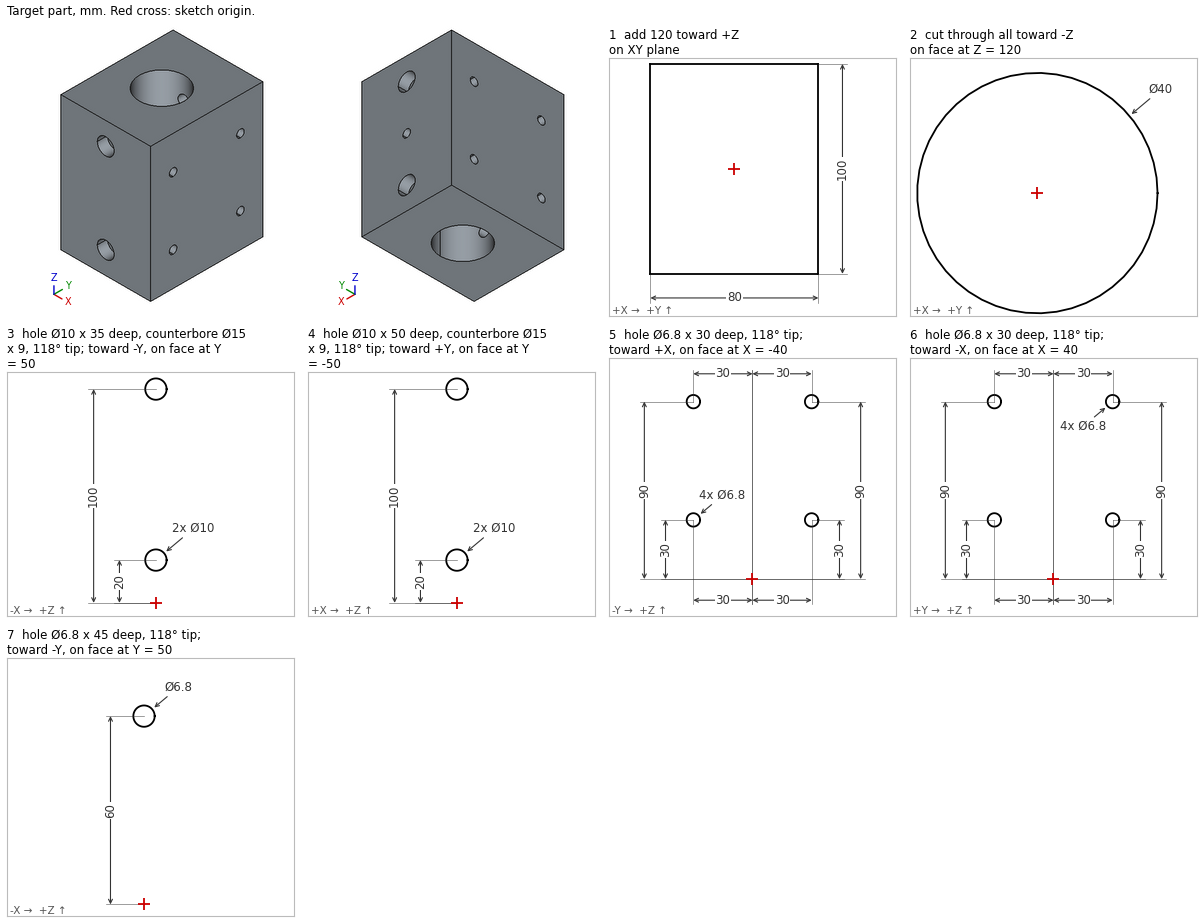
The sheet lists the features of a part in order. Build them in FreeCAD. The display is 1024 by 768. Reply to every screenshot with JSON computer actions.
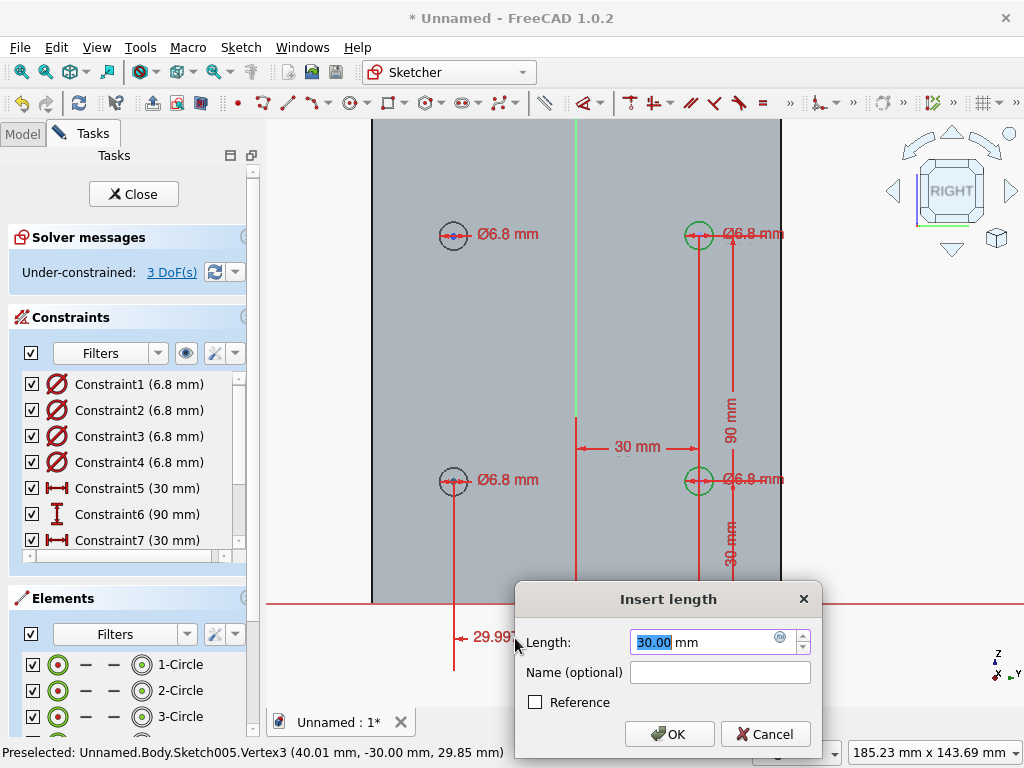
{"action": "type", "text": "30"}
{"action": "key", "text": "Return"}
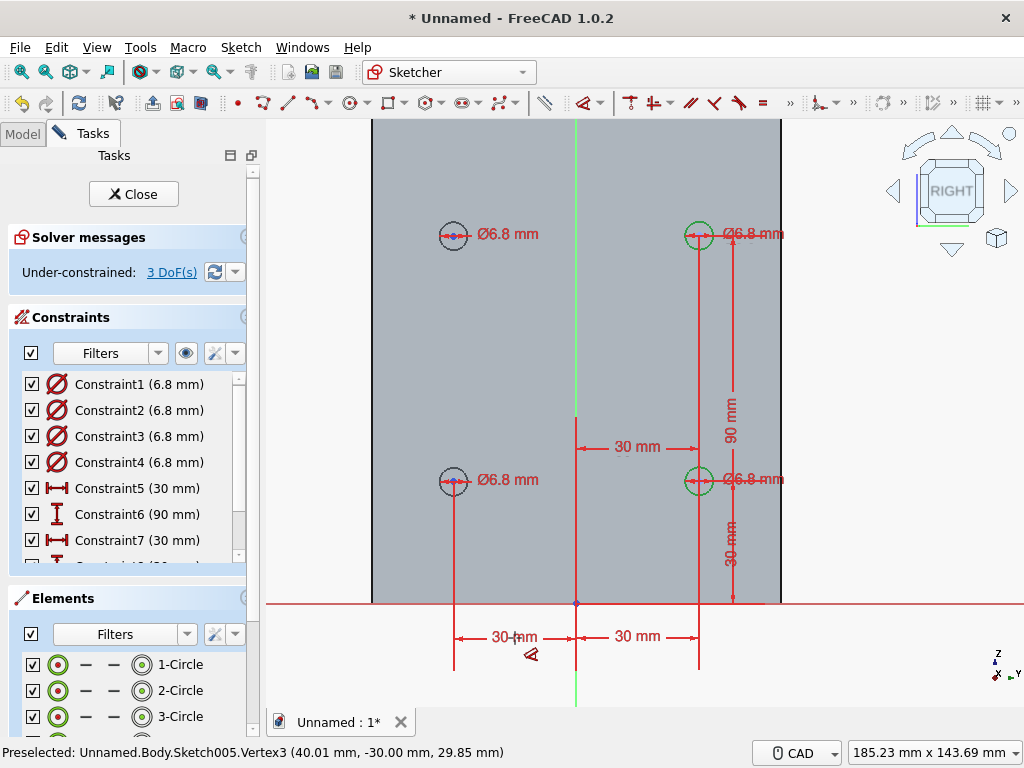
{"action": "left_click", "coordinate": [454, 482]}
{"action": "left_click", "coordinate": [420, 543]}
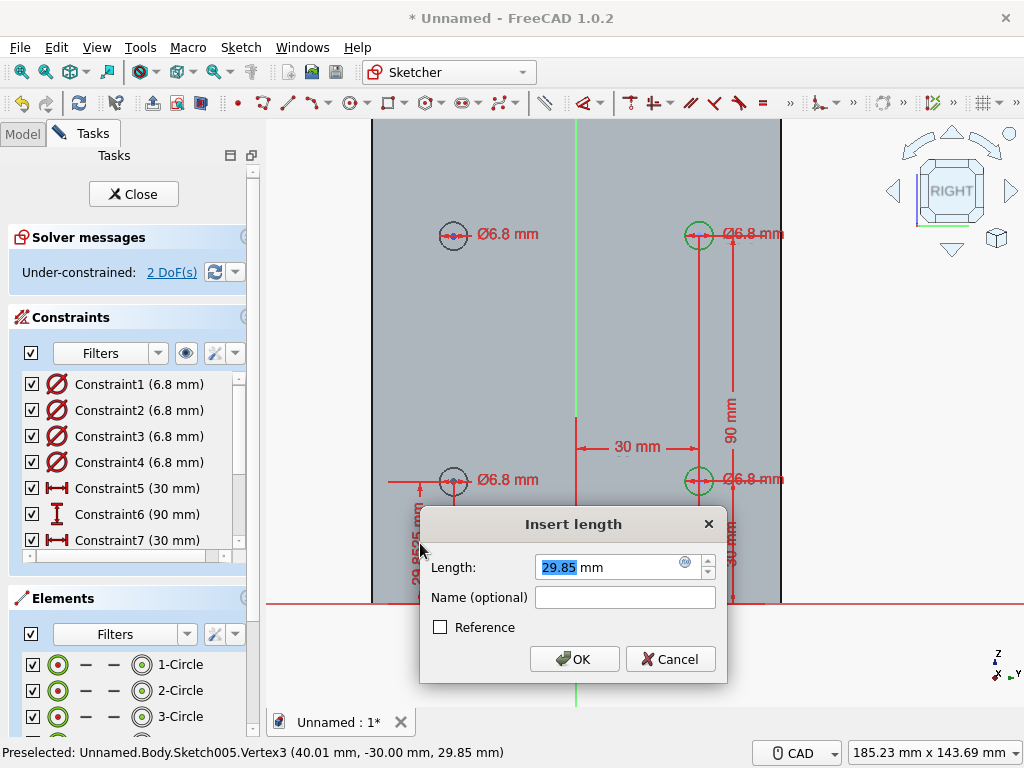
{"action": "type", "text": "30"}
{"action": "key", "text": "Return"}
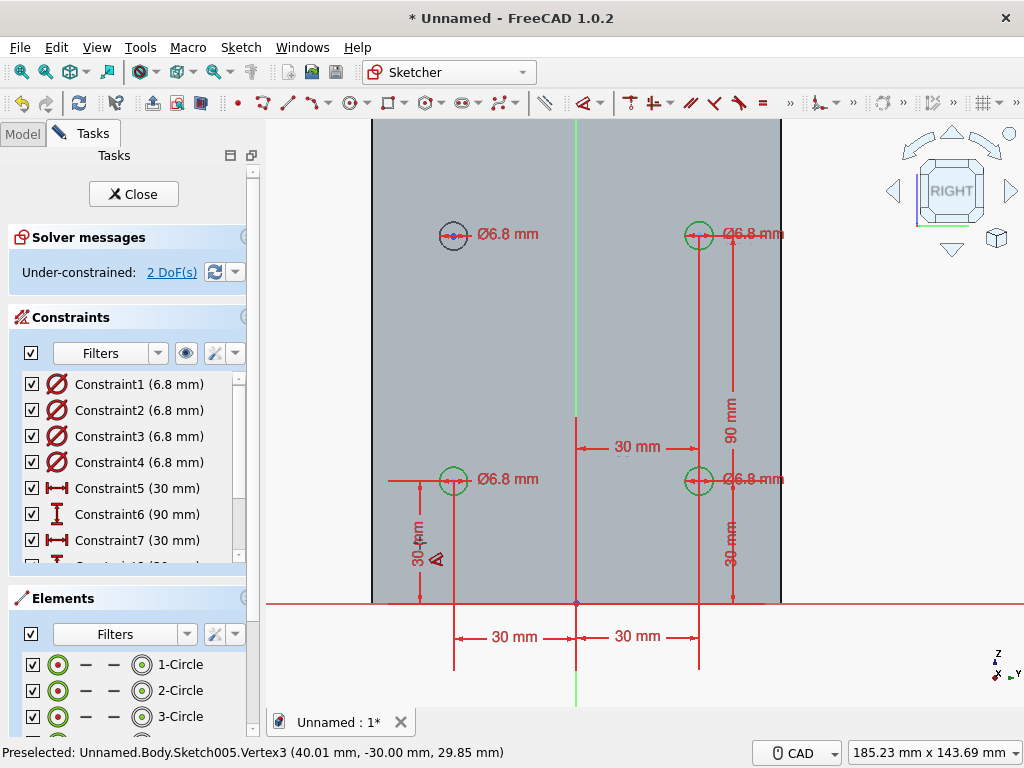
{"action": "left_click", "coordinate": [454, 236]}
{"action": "left_click", "coordinate": [515, 202]}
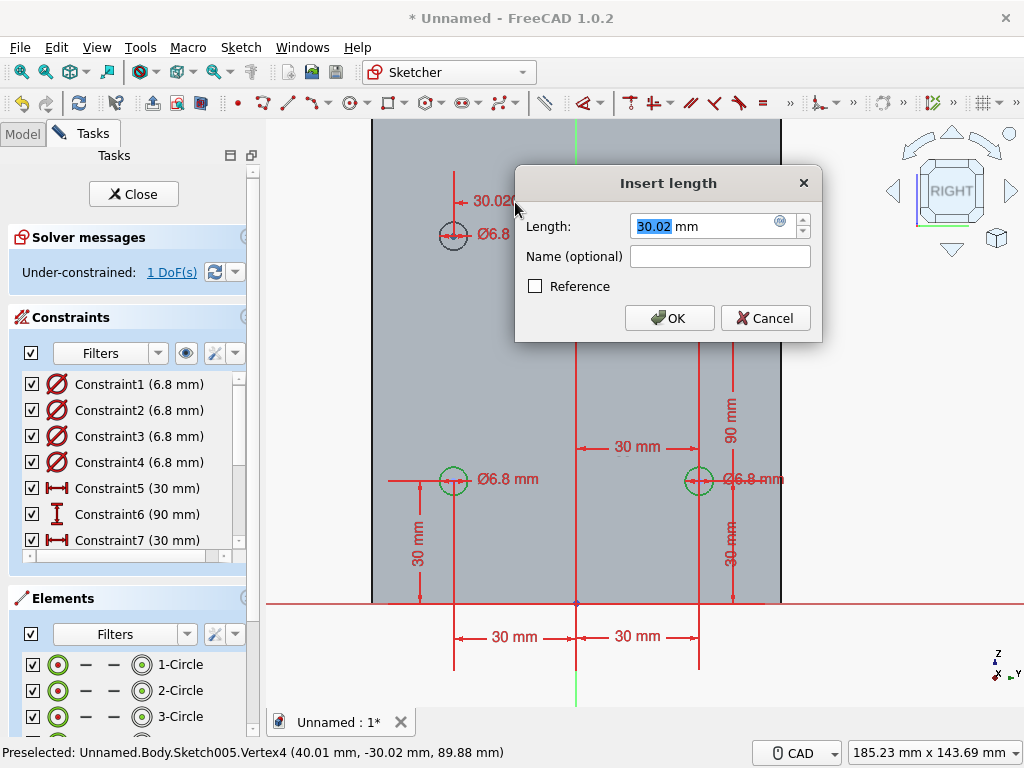
{"action": "type", "text": "30"}
{"action": "key", "text": "Return"}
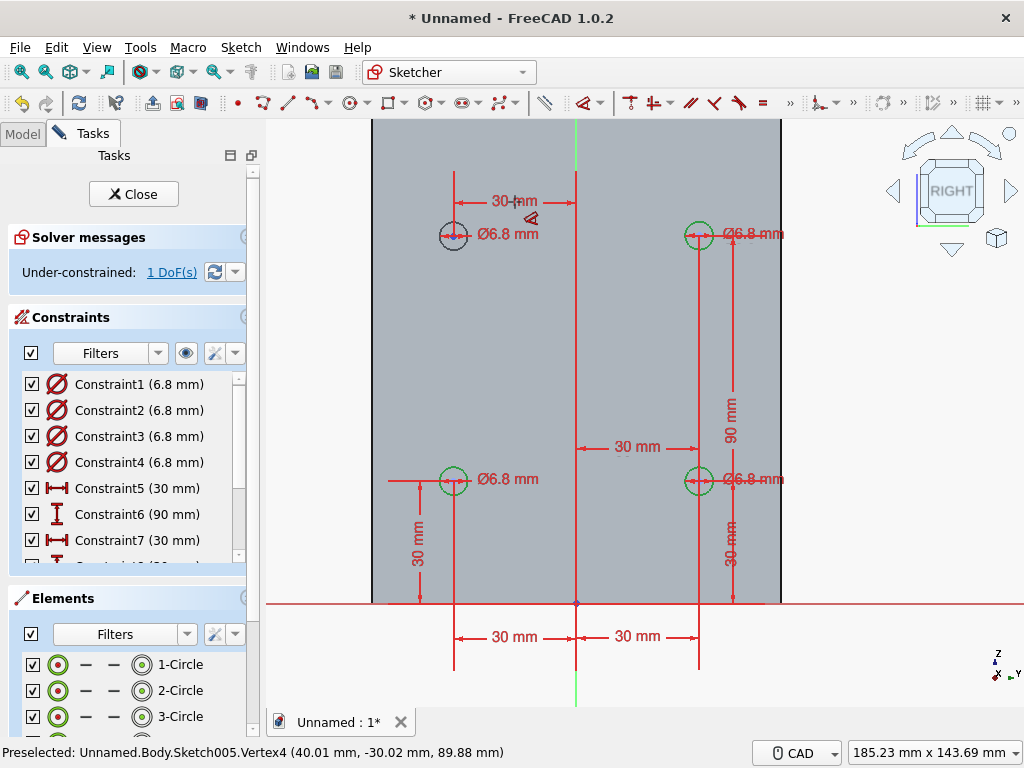
{"action": "left_click", "coordinate": [454, 236]}
{"action": "left_click", "coordinate": [420, 420]}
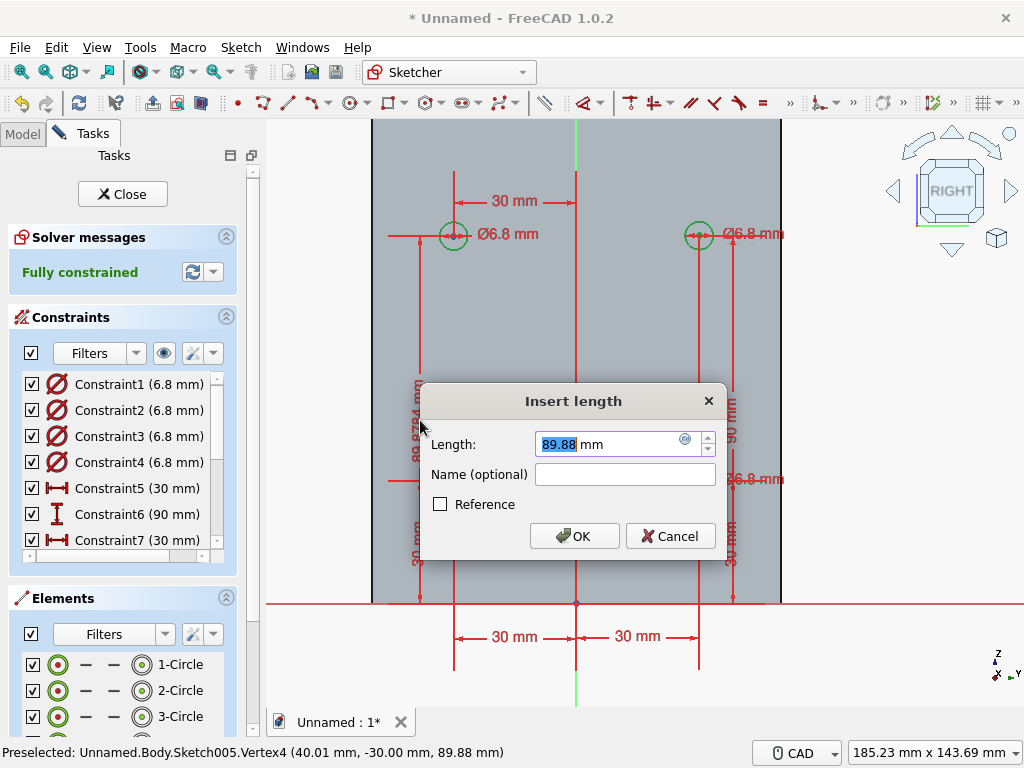
{"action": "type", "text": "90"}
{"action": "key", "text": "Return"}
{"action": "key", "text": "Escape"}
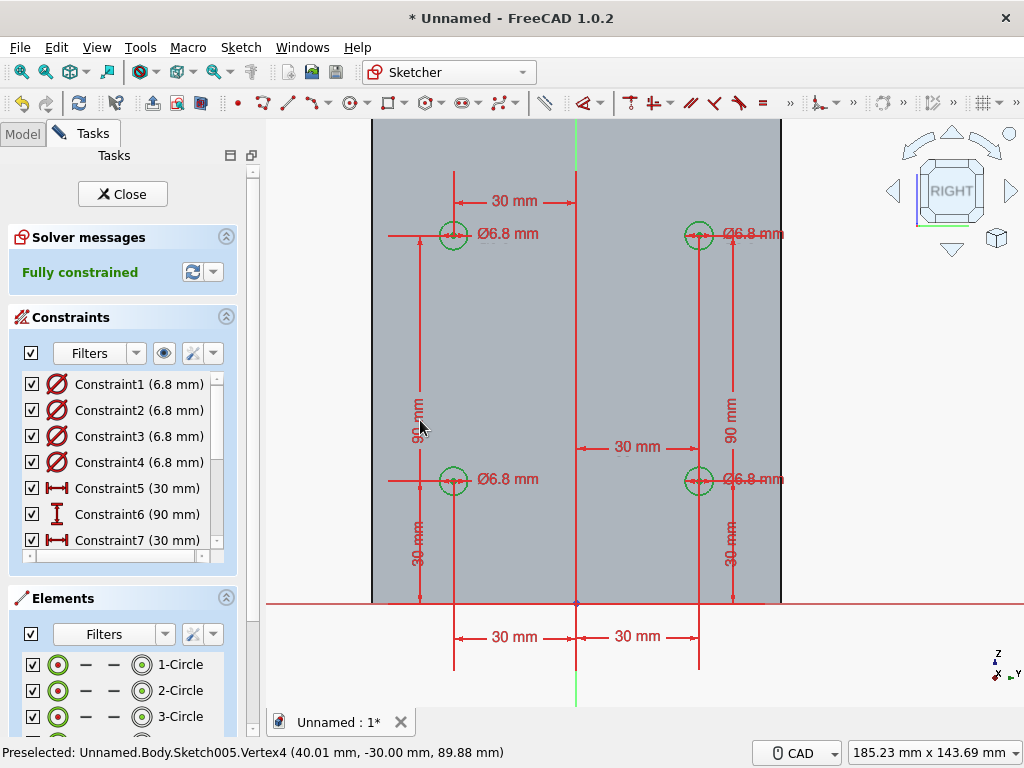
{"action": "left_click", "coordinate": [123, 194]}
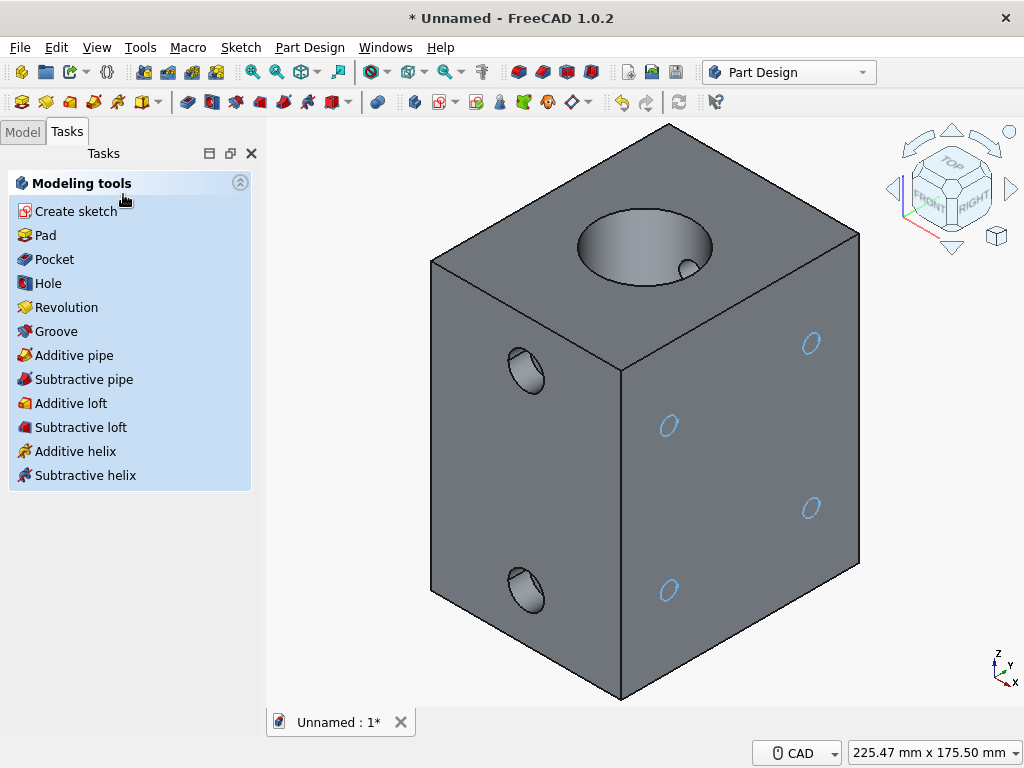
{"action": "left_click", "coordinate": [212, 102]}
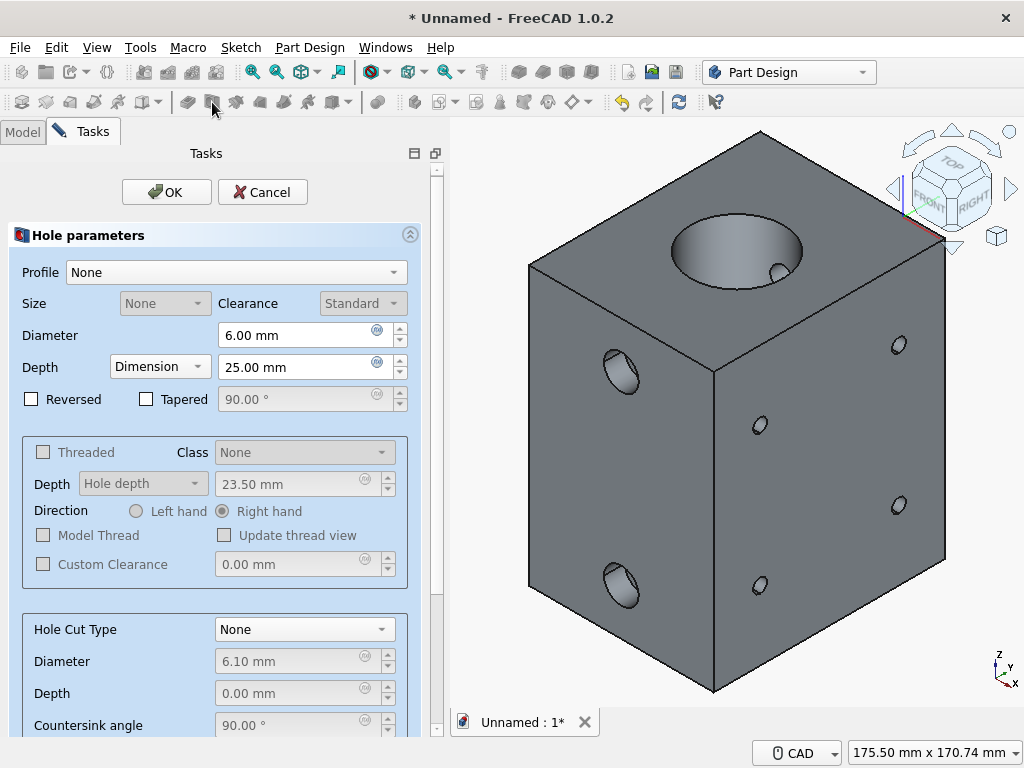
{"action": "triple_click", "coordinate": [305, 335]}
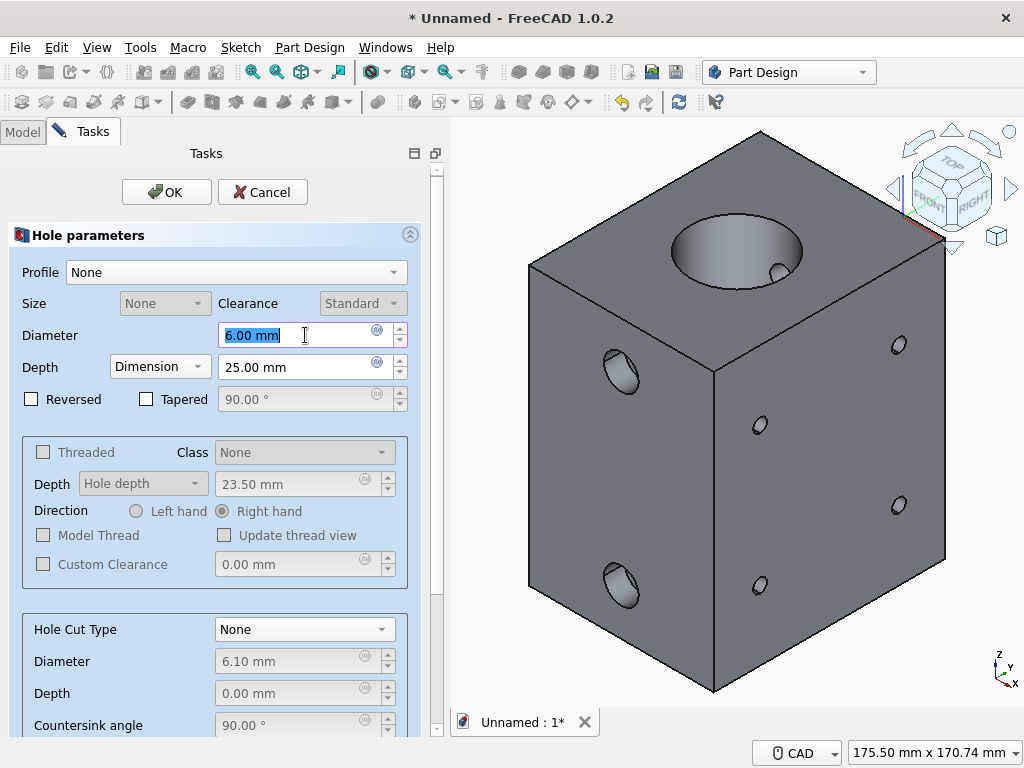
{"action": "type", "text": "6.8"}
{"action": "key", "text": "Tab"}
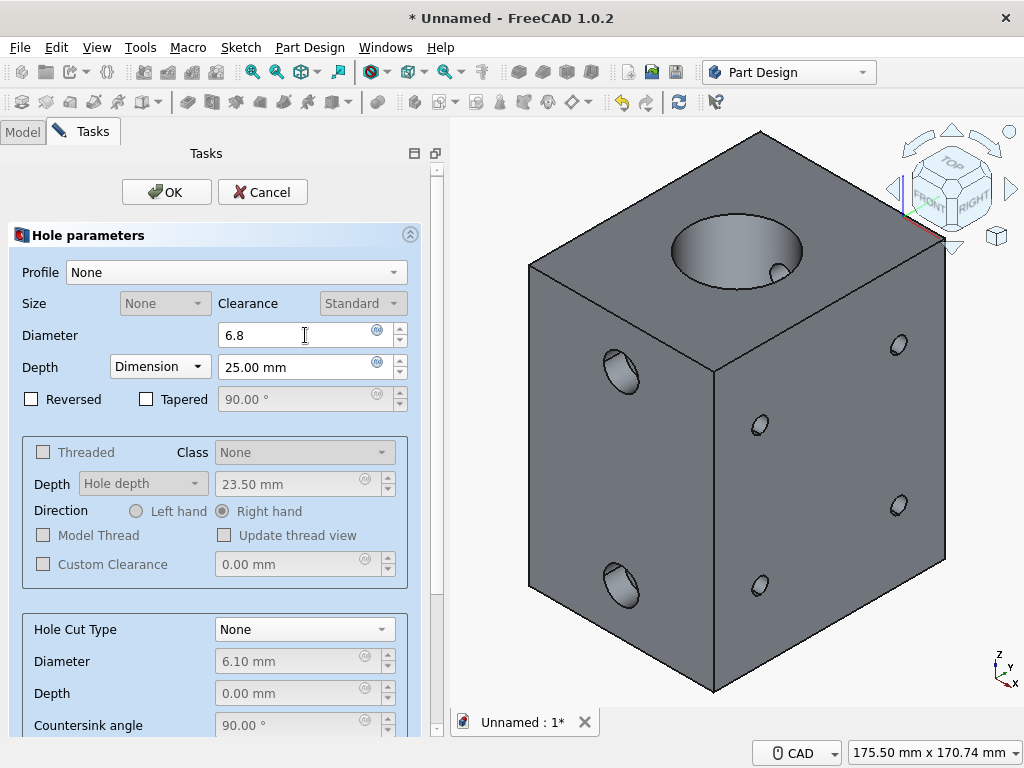
{"action": "triple_click", "coordinate": [305, 367]}